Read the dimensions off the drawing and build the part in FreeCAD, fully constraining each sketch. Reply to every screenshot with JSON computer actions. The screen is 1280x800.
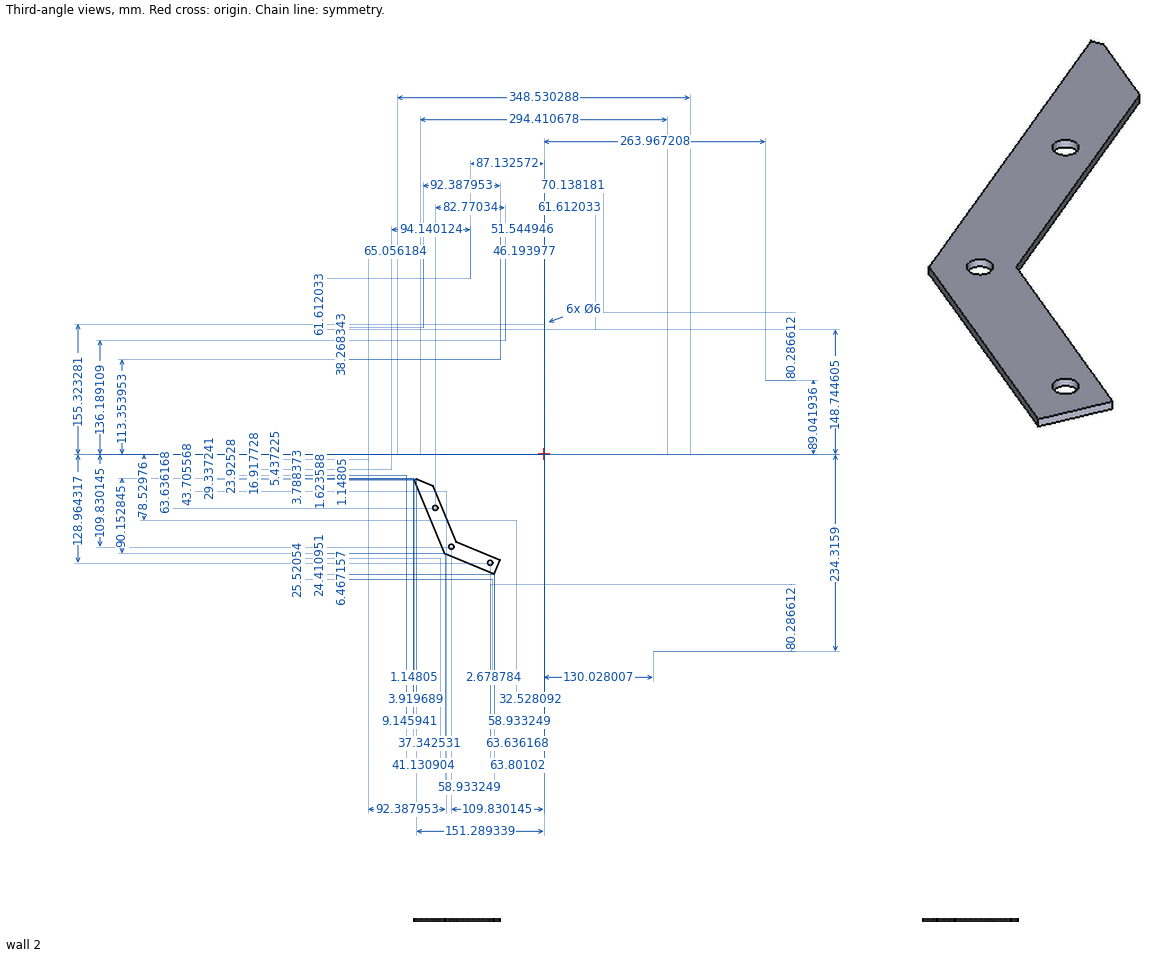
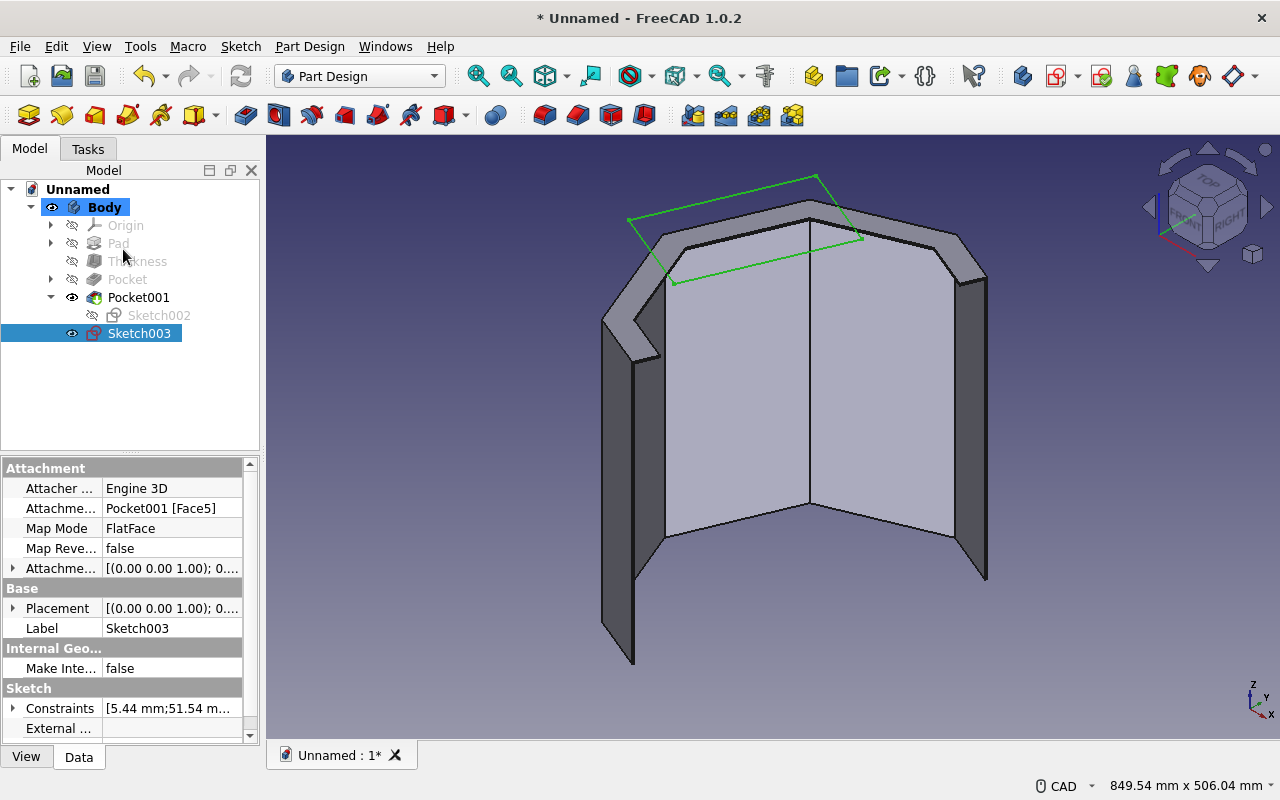
{"action": "left_click", "coordinate": [246, 116]}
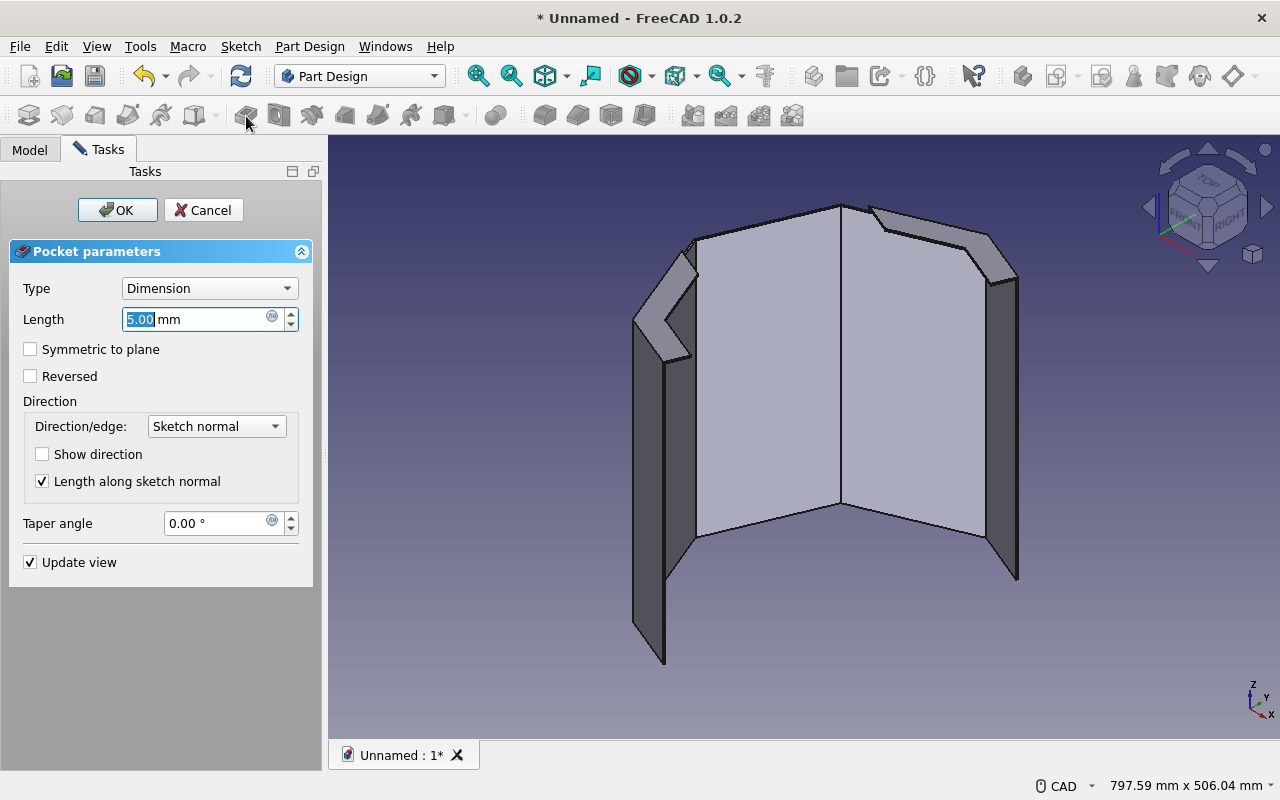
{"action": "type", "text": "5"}
{"action": "key", "text": "Tab"}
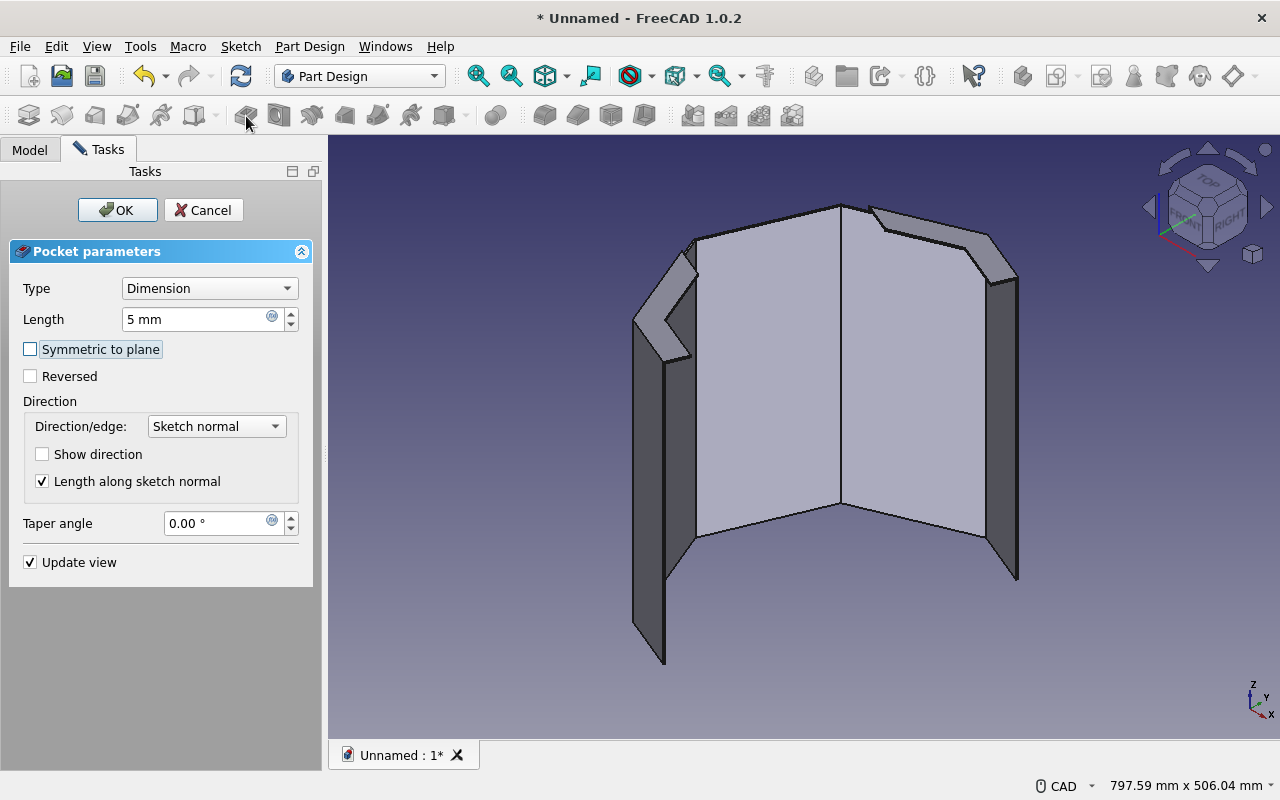
{"action": "left_click", "coordinate": [118, 210]}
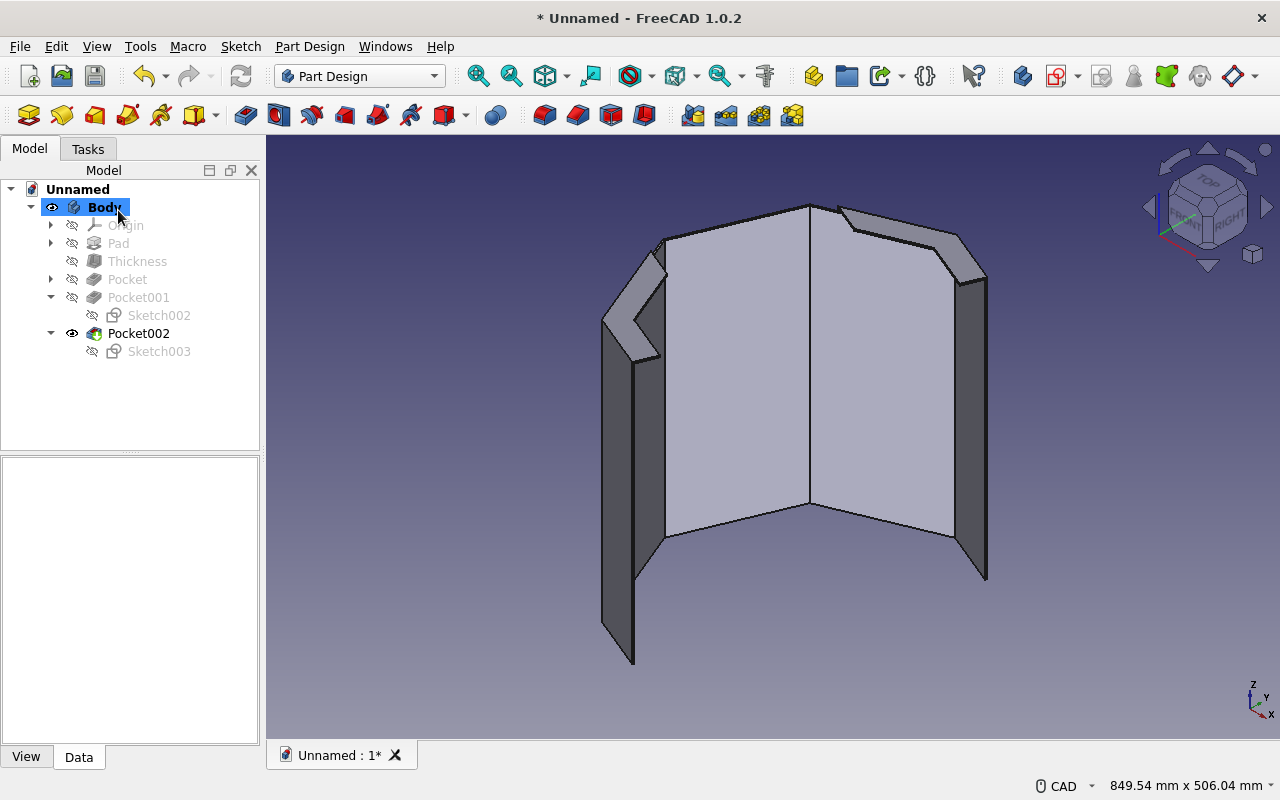
{"action": "left_click", "coordinate": [924, 234]}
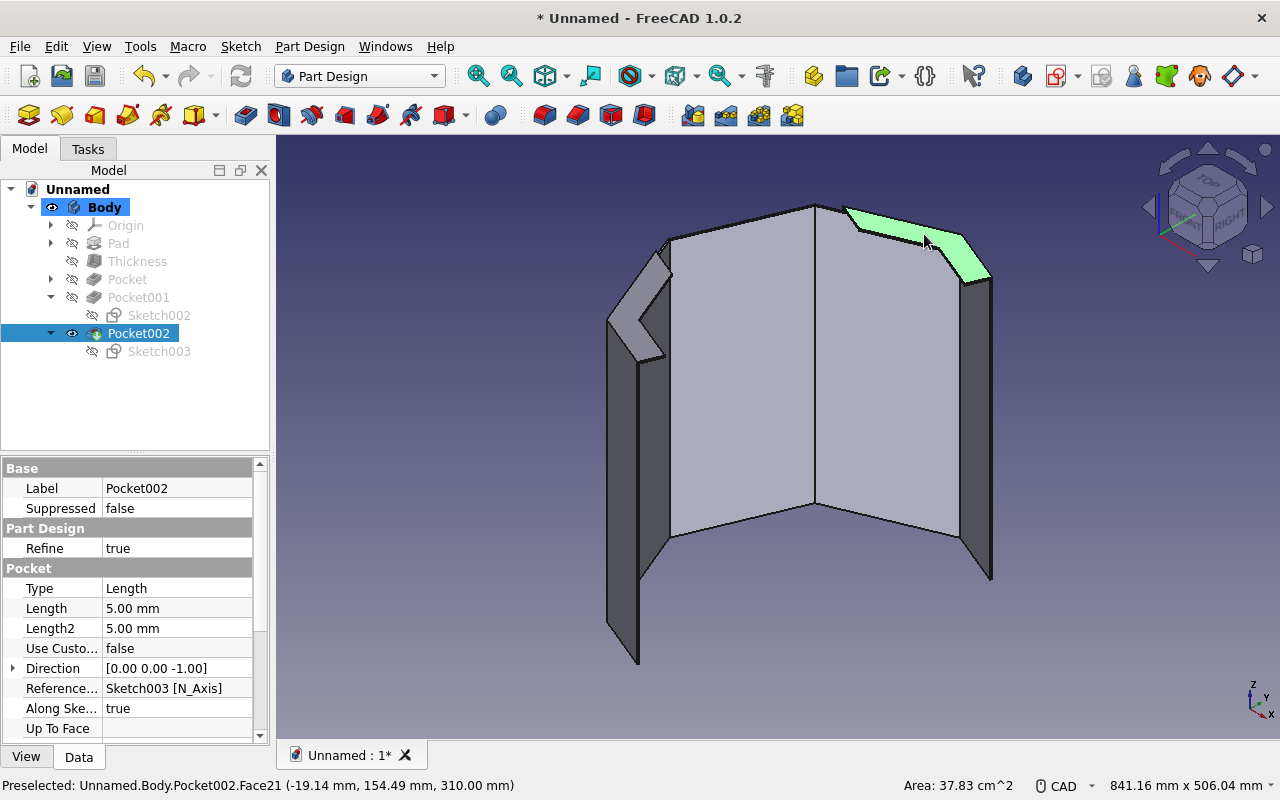
{"action": "left_click", "coordinate": [1056, 76]}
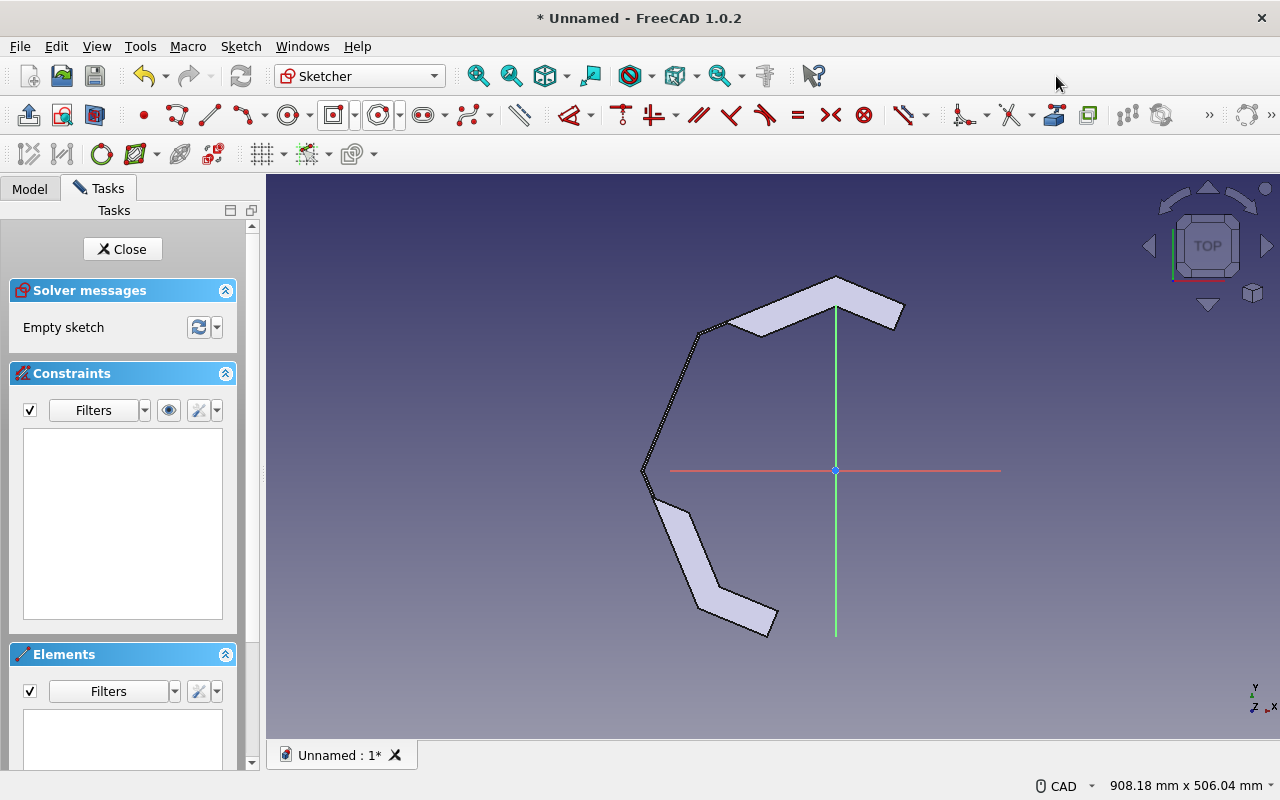
{"action": "left_click", "coordinate": [288, 116]}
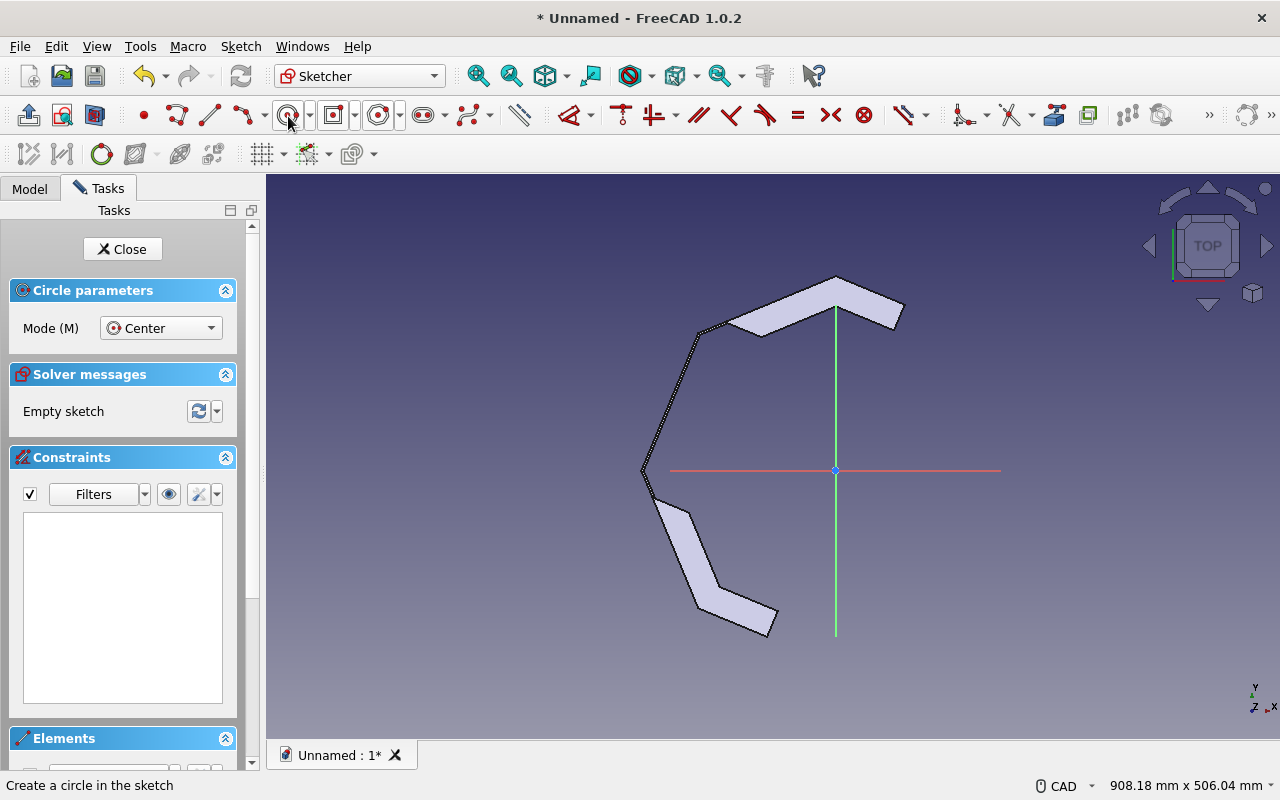
{"action": "scroll", "coordinate": [836, 297], "scroll_direction": "up", "scroll_amount": 10}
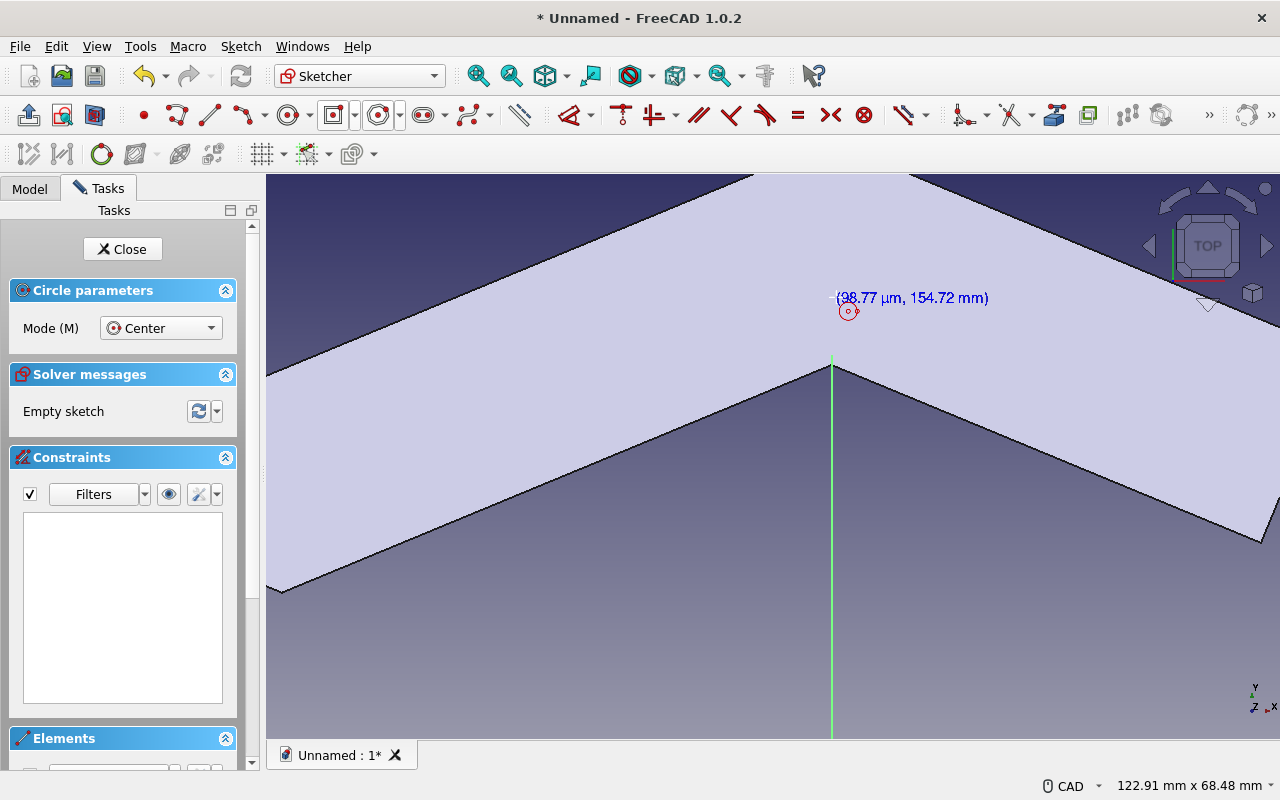
{"action": "scroll", "coordinate": [747, 256], "scroll_direction": "down", "scroll_amount": 9}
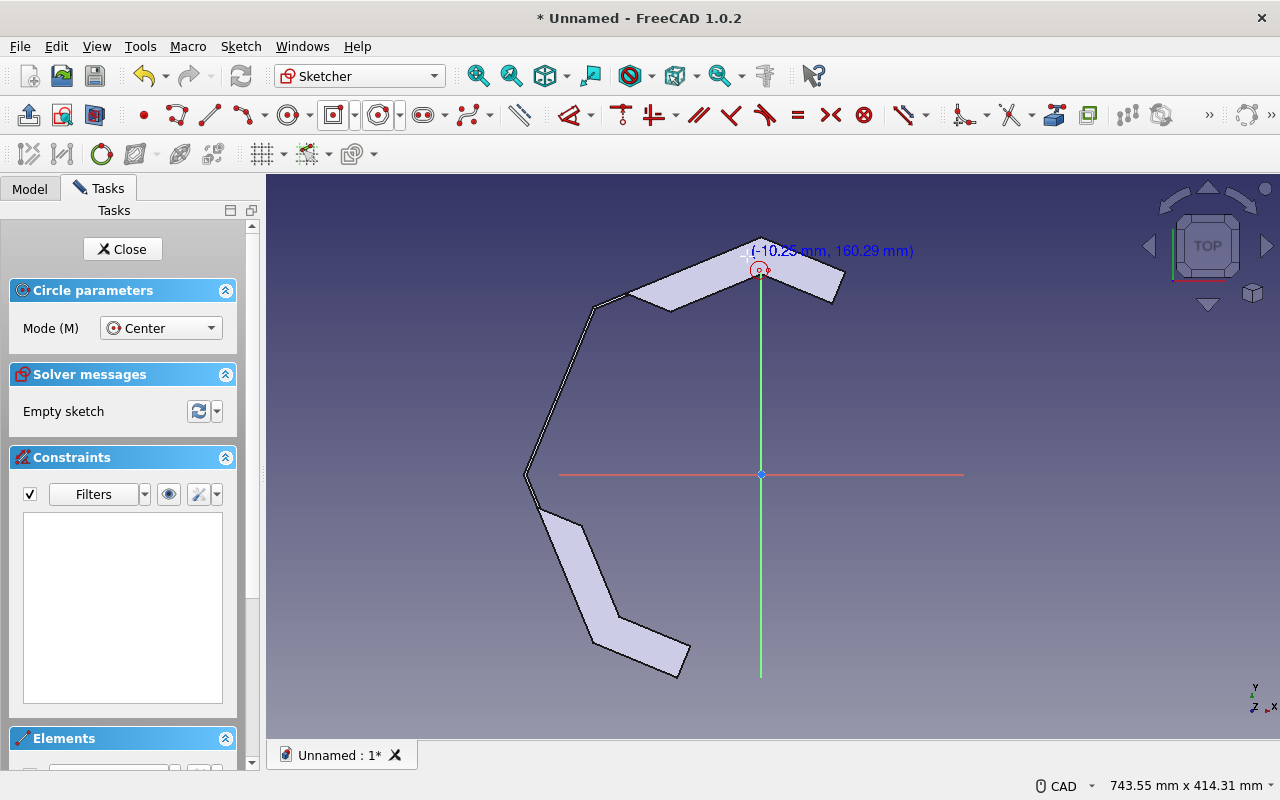
{"action": "left_click", "coordinate": [761, 263]}